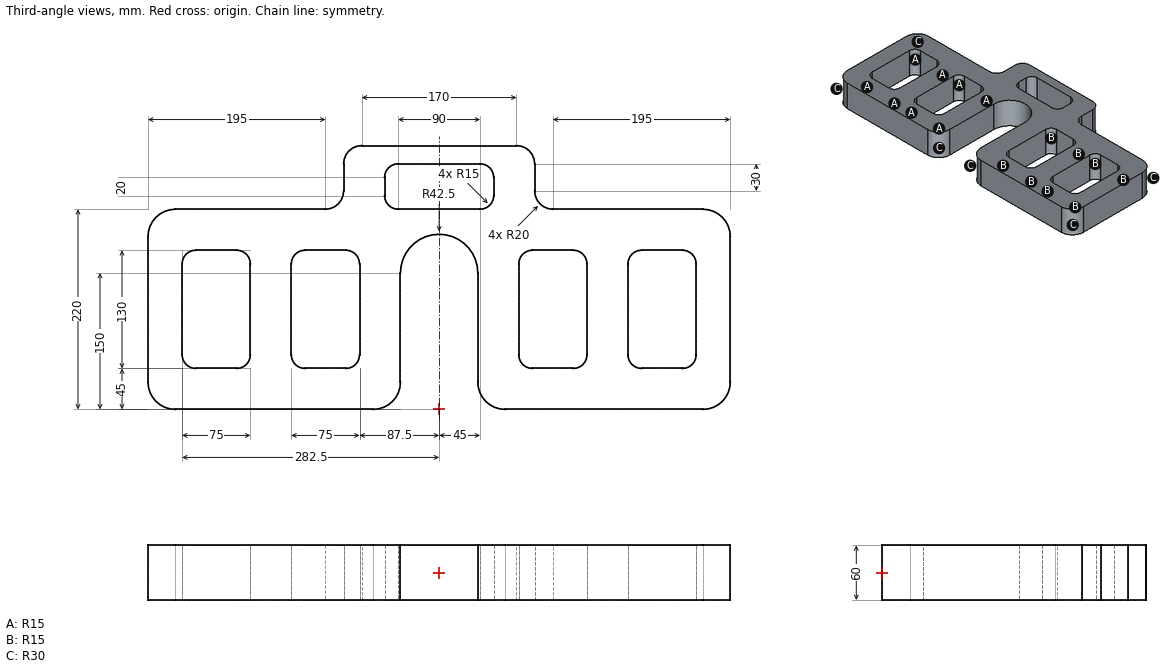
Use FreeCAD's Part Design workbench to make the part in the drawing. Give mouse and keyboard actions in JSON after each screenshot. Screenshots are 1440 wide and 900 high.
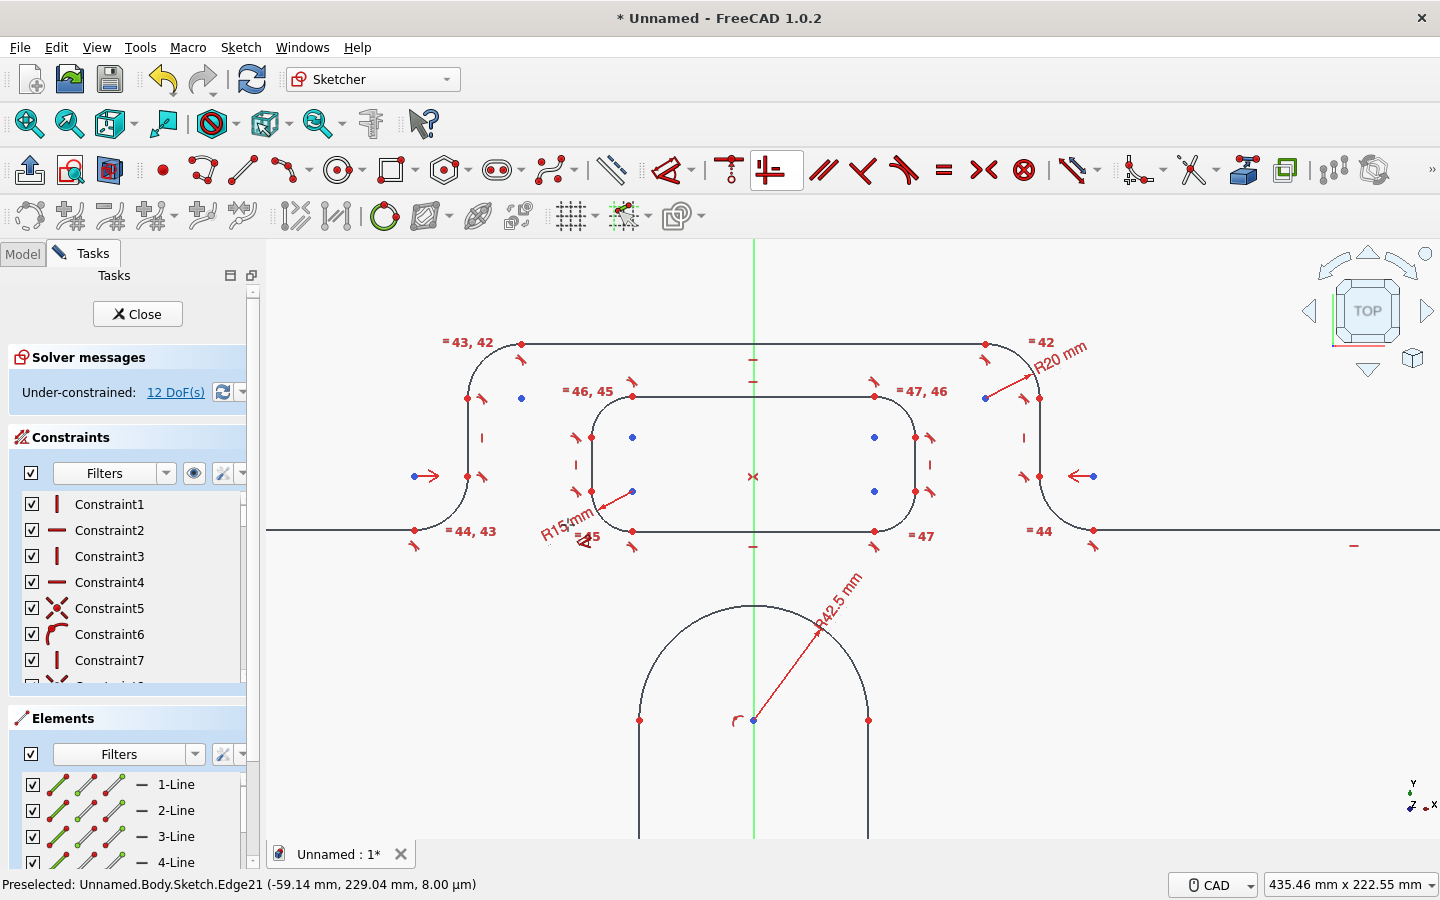
{"action": "left_click", "coordinate": [1040, 453]}
{"action": "left_click", "coordinate": [1074, 437]}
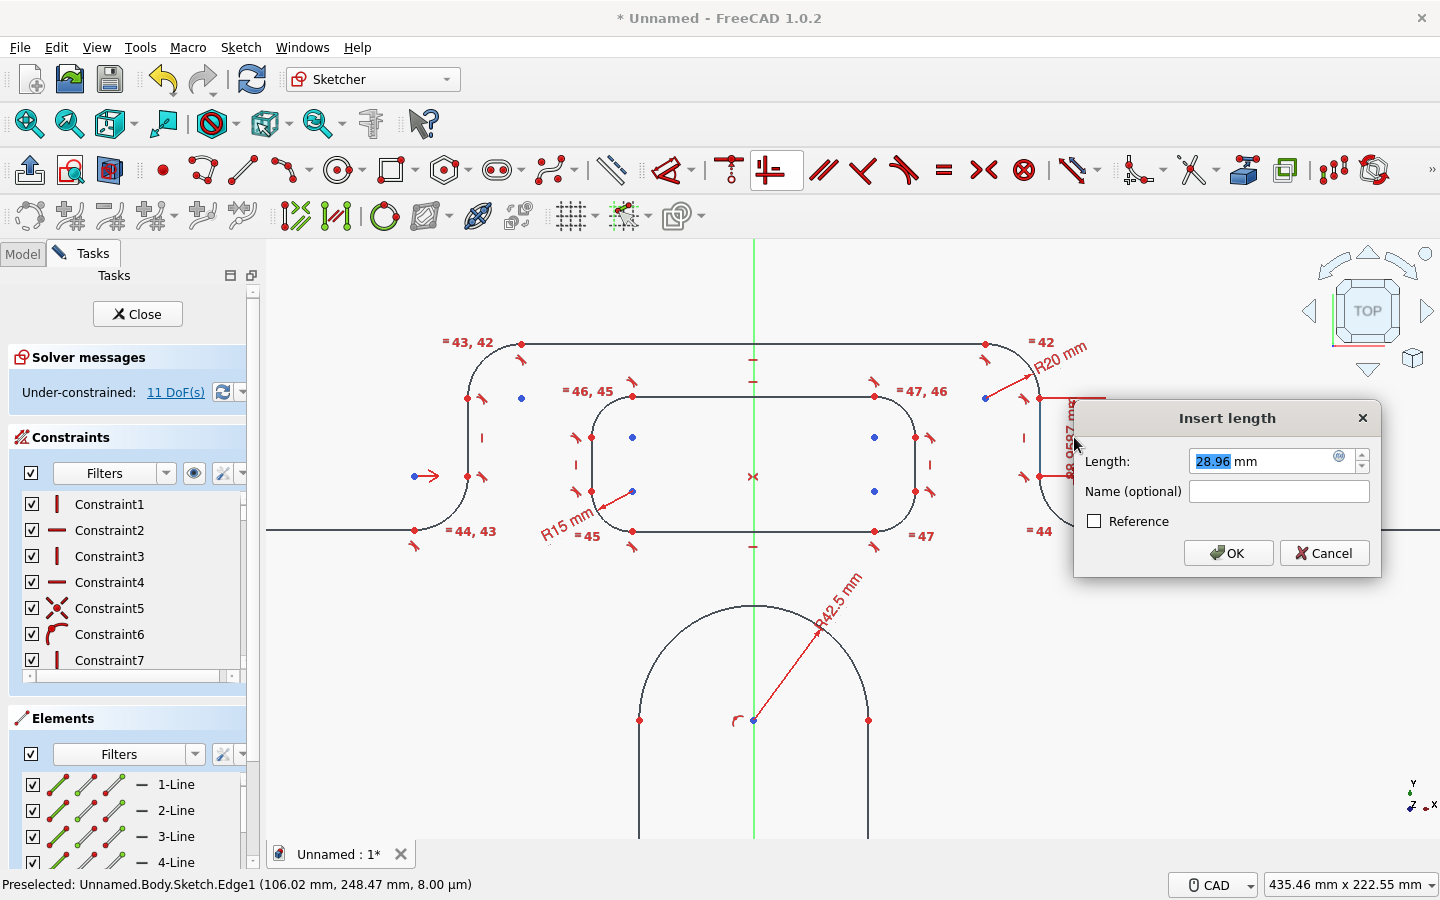
{"action": "type", "text": "30"}
{"action": "key", "text": "Return"}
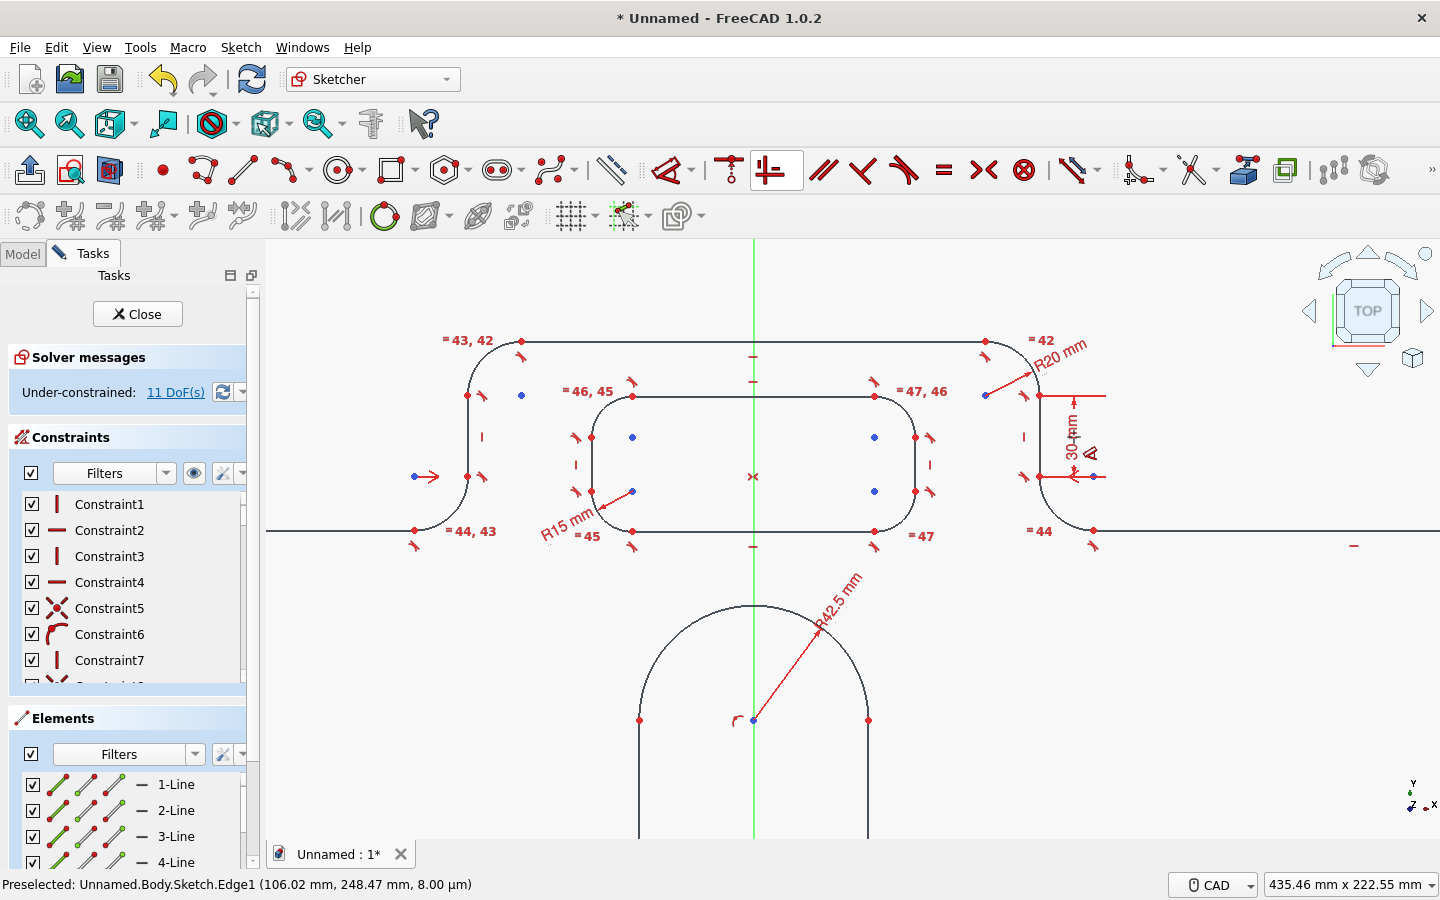
{"action": "left_click", "coordinate": [802, 532]}
{"action": "left_click", "coordinate": [698, 498]}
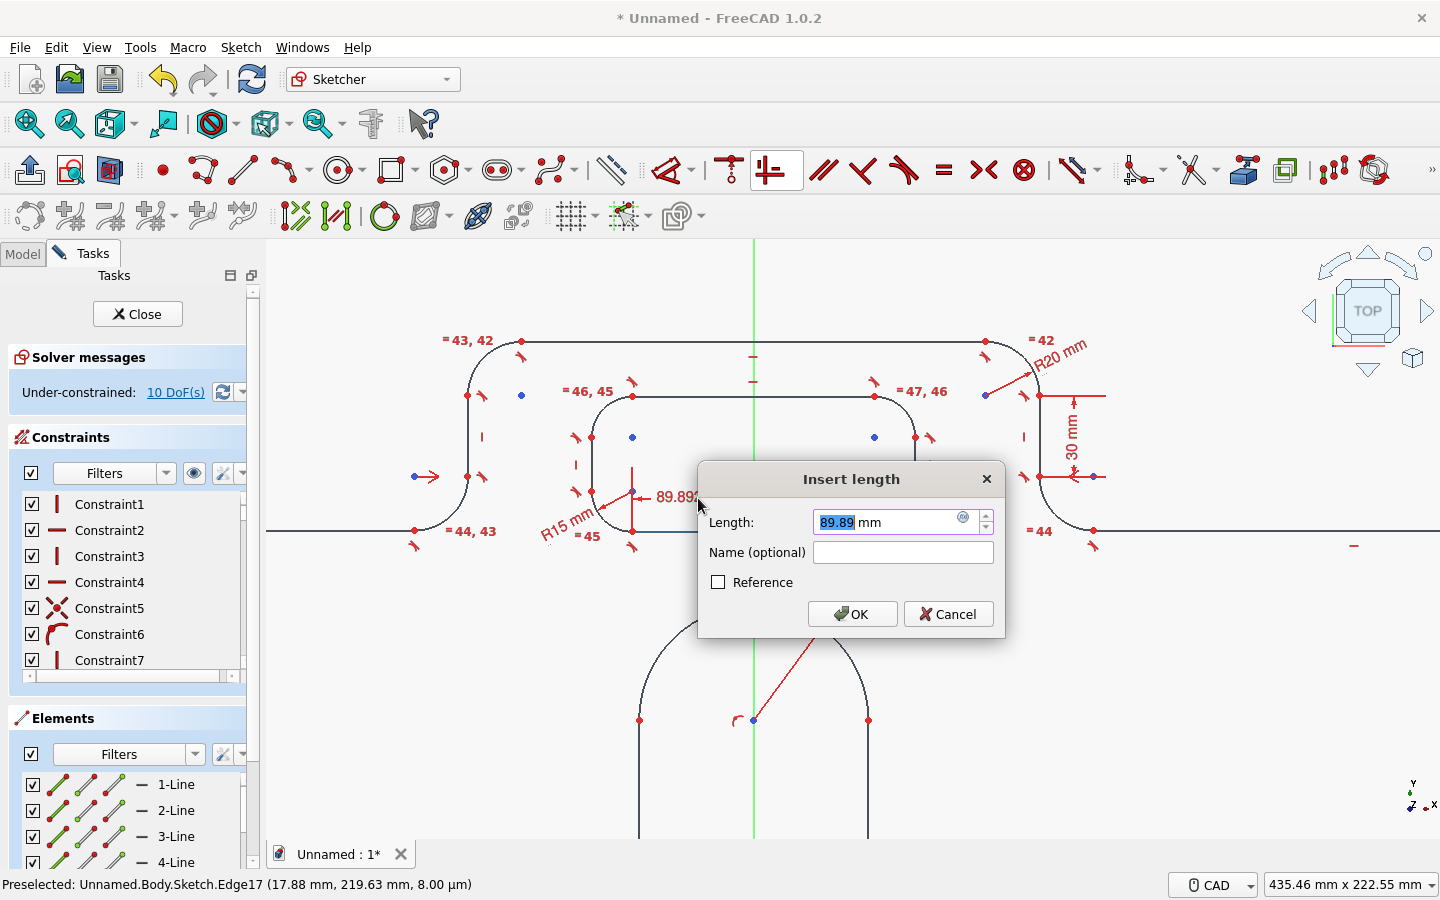
{"action": "type", "text": "90"}
{"action": "key", "text": "Return"}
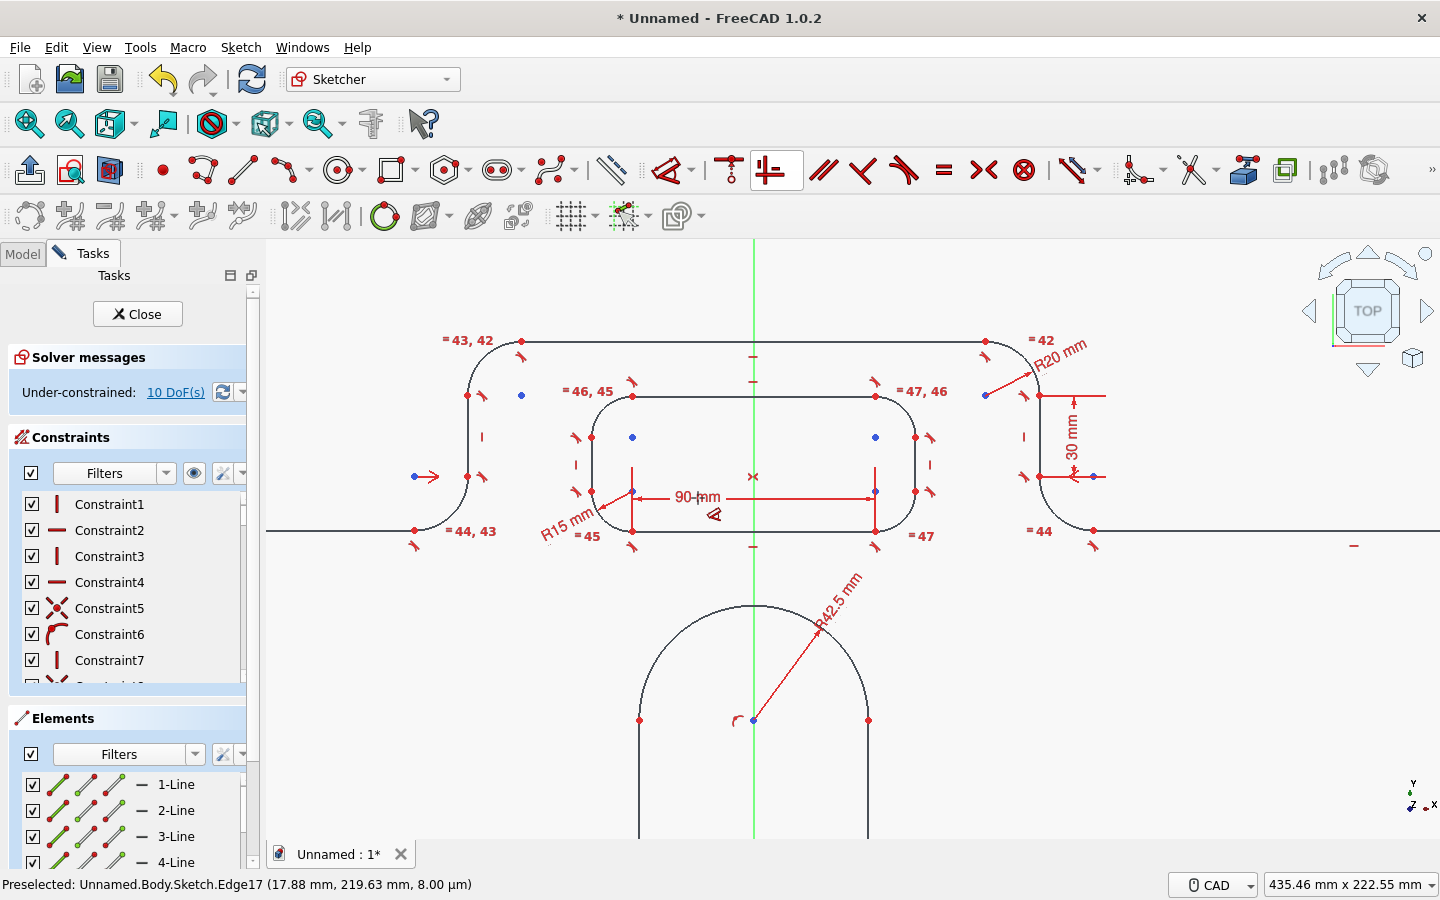
{"action": "left_click", "coordinate": [592, 475]}
{"action": "left_click", "coordinate": [558, 464]}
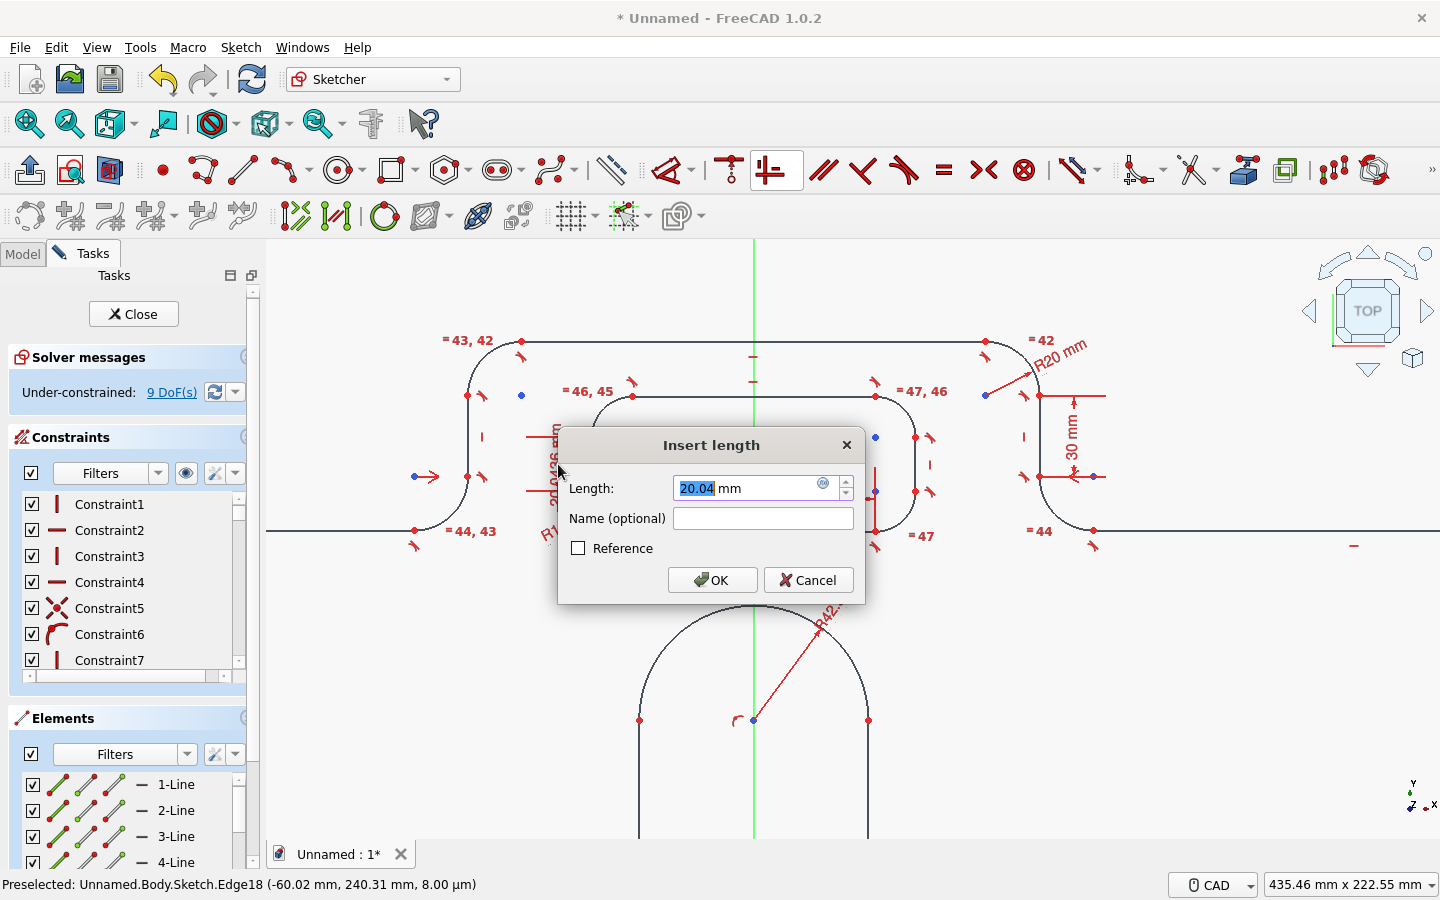
{"action": "type", "text": "20"}
{"action": "key", "text": "Return"}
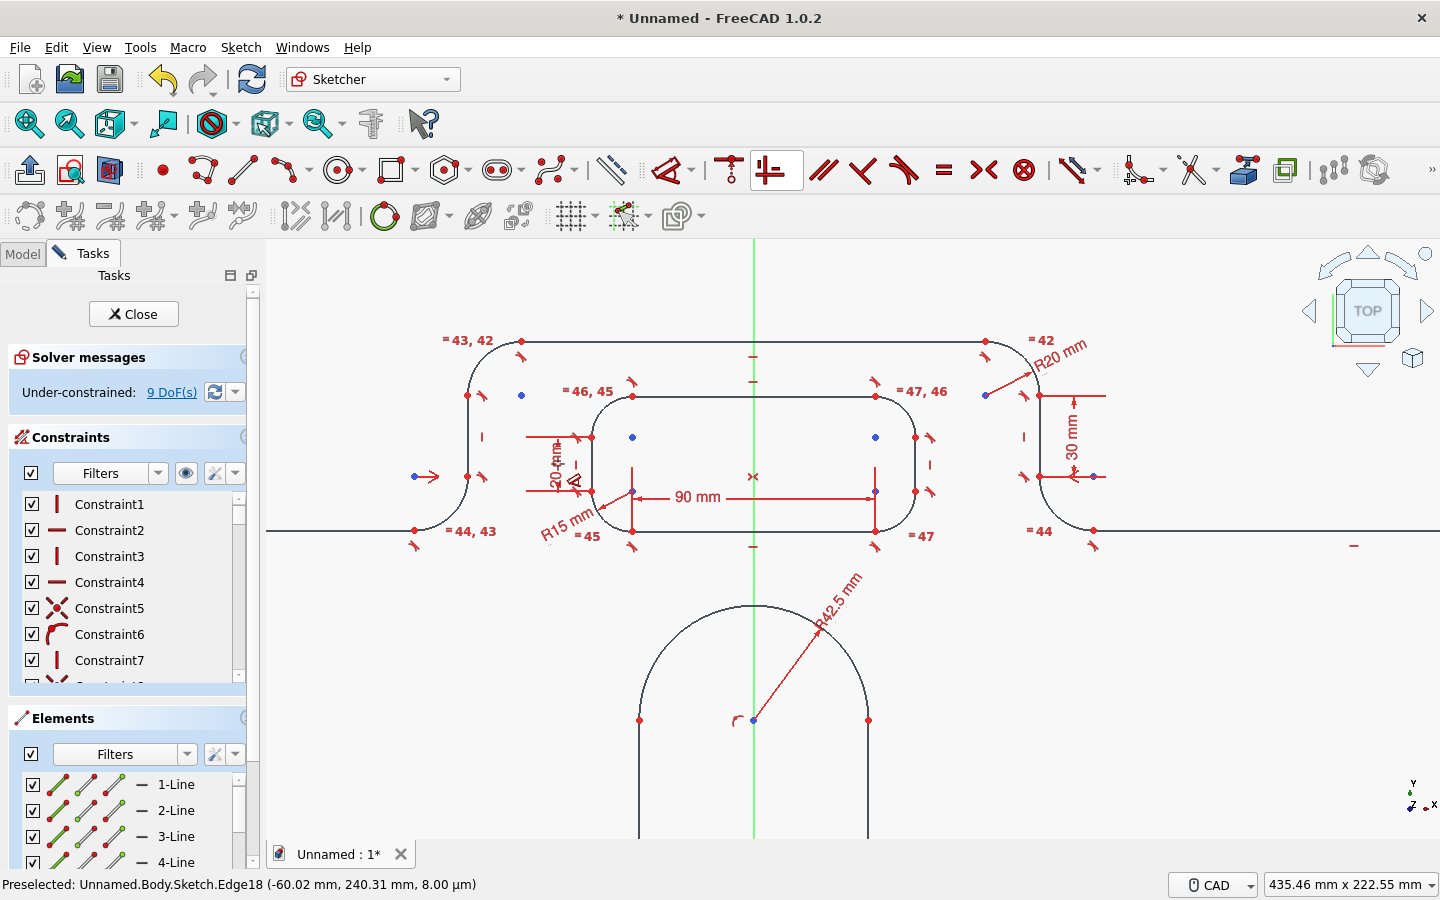
{"action": "left_click", "coordinate": [847, 342]}
{"action": "left_click", "coordinate": [647, 308]}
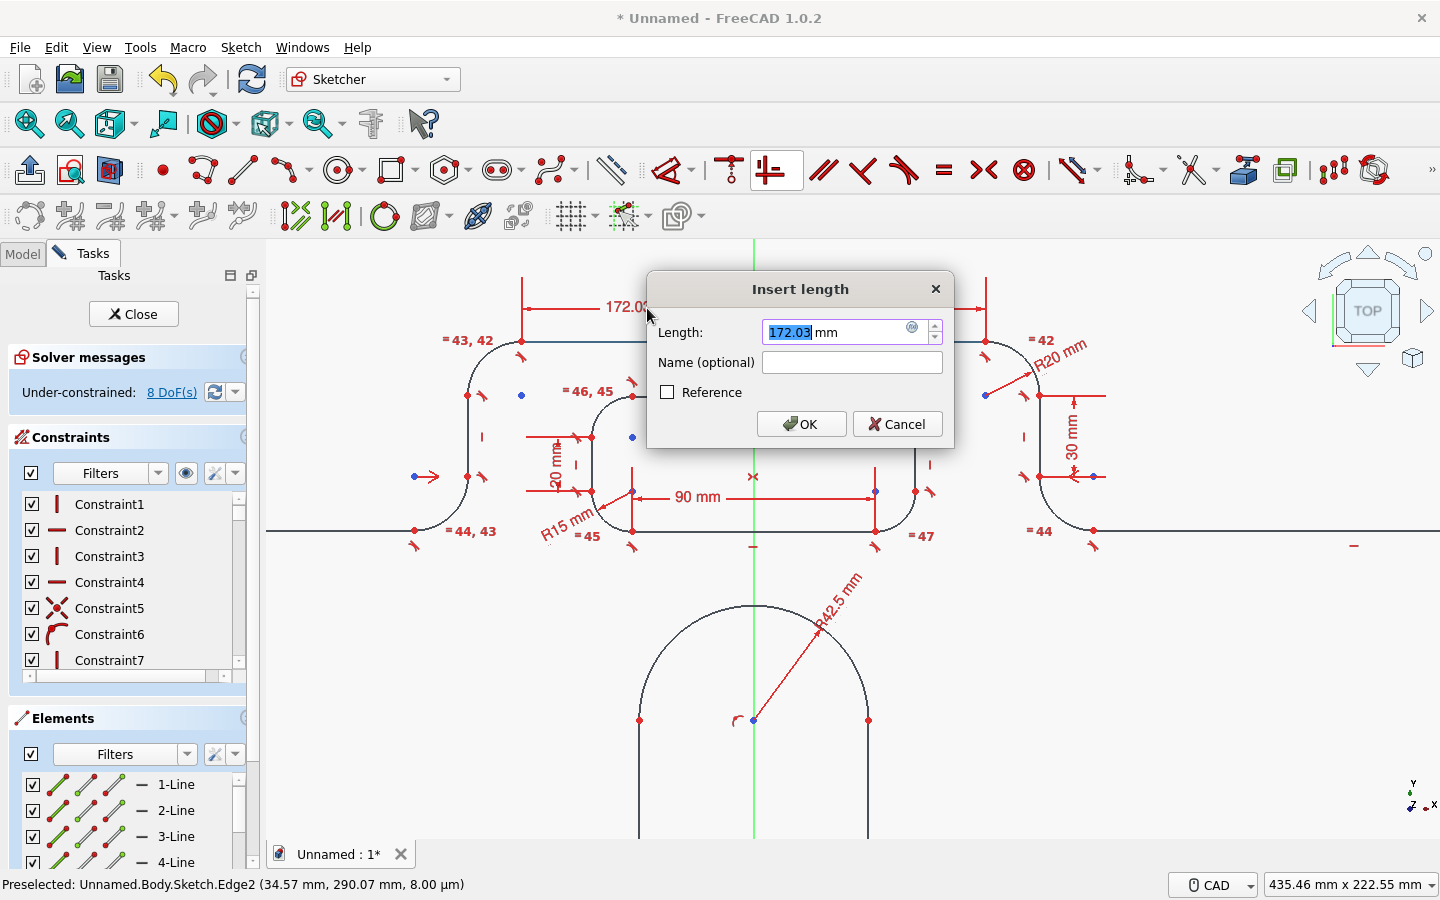
{"action": "type", "text": "170"}
{"action": "key", "text": "Return"}